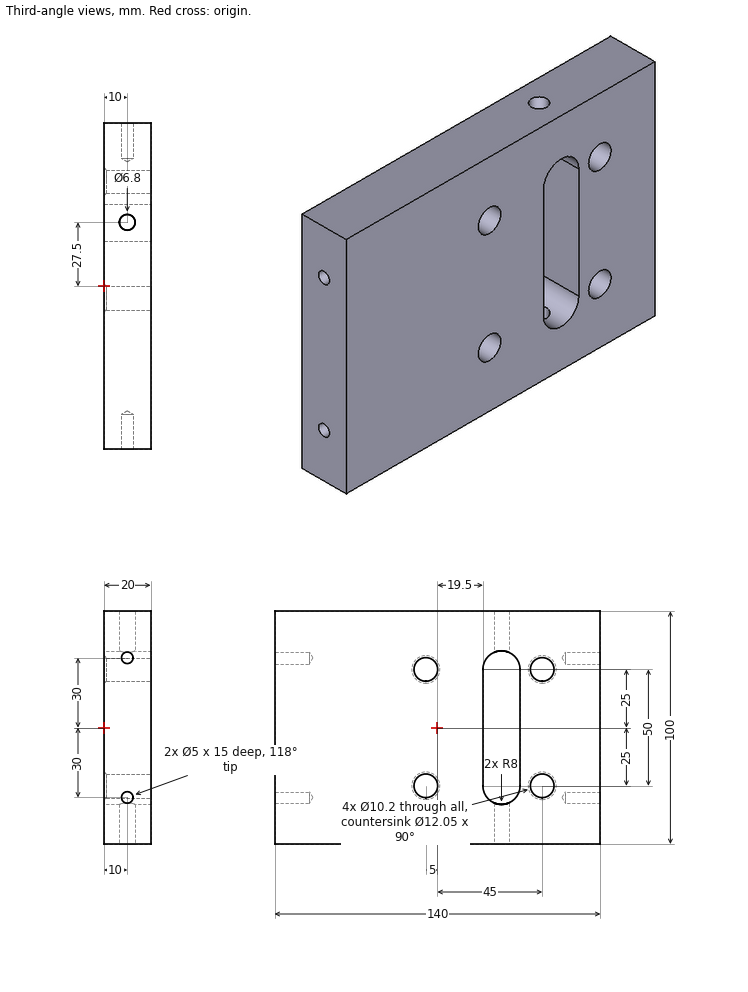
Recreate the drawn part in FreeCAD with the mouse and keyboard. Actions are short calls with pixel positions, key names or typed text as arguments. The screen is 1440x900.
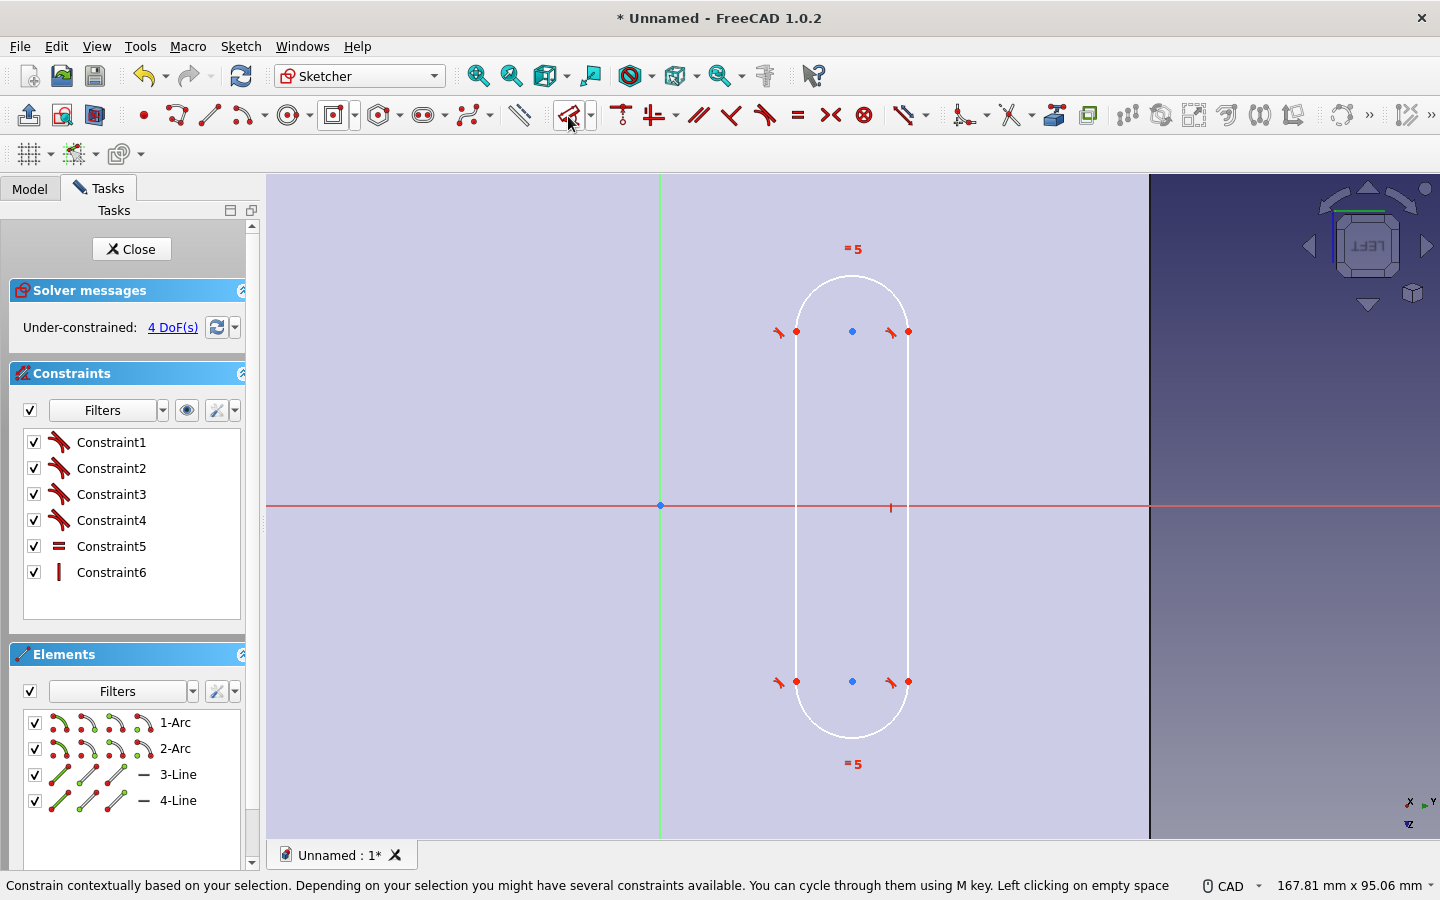
click(819, 727)
click(800, 753)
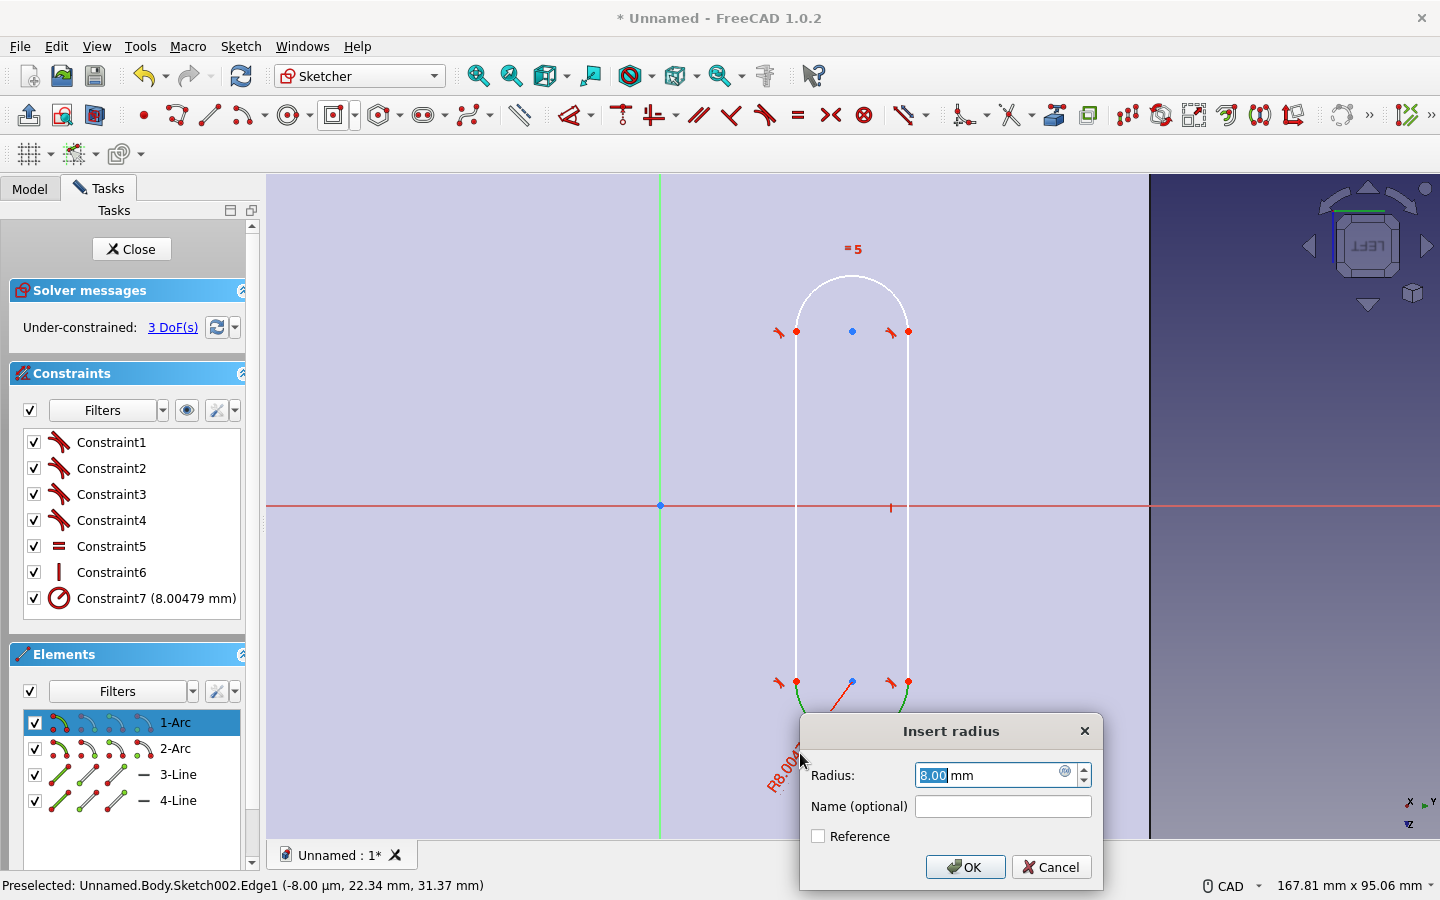
text(8)
key(Return)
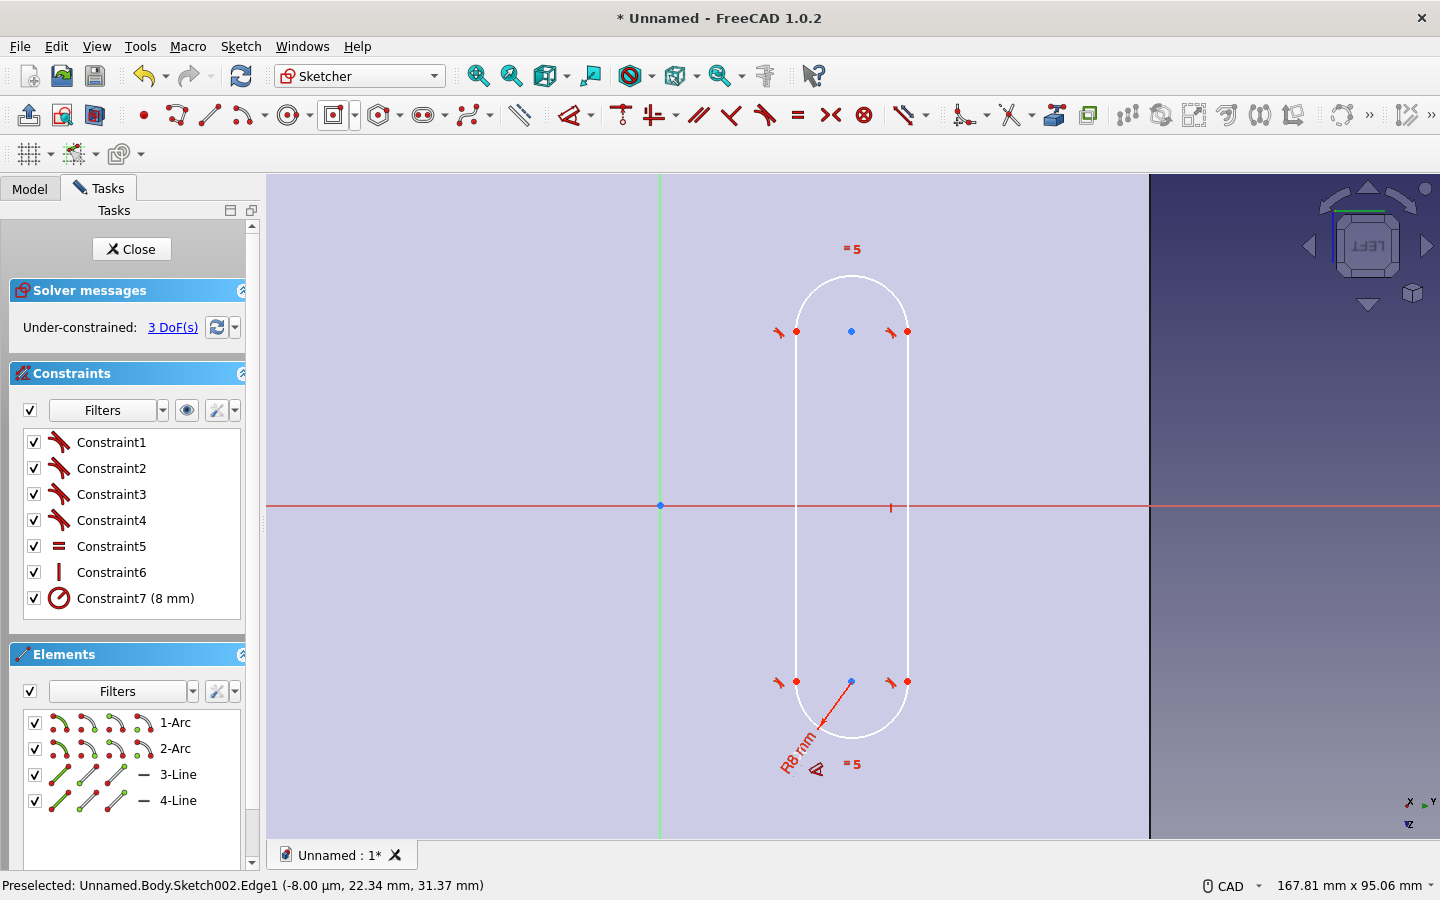
click(796, 577)
click(830, 427)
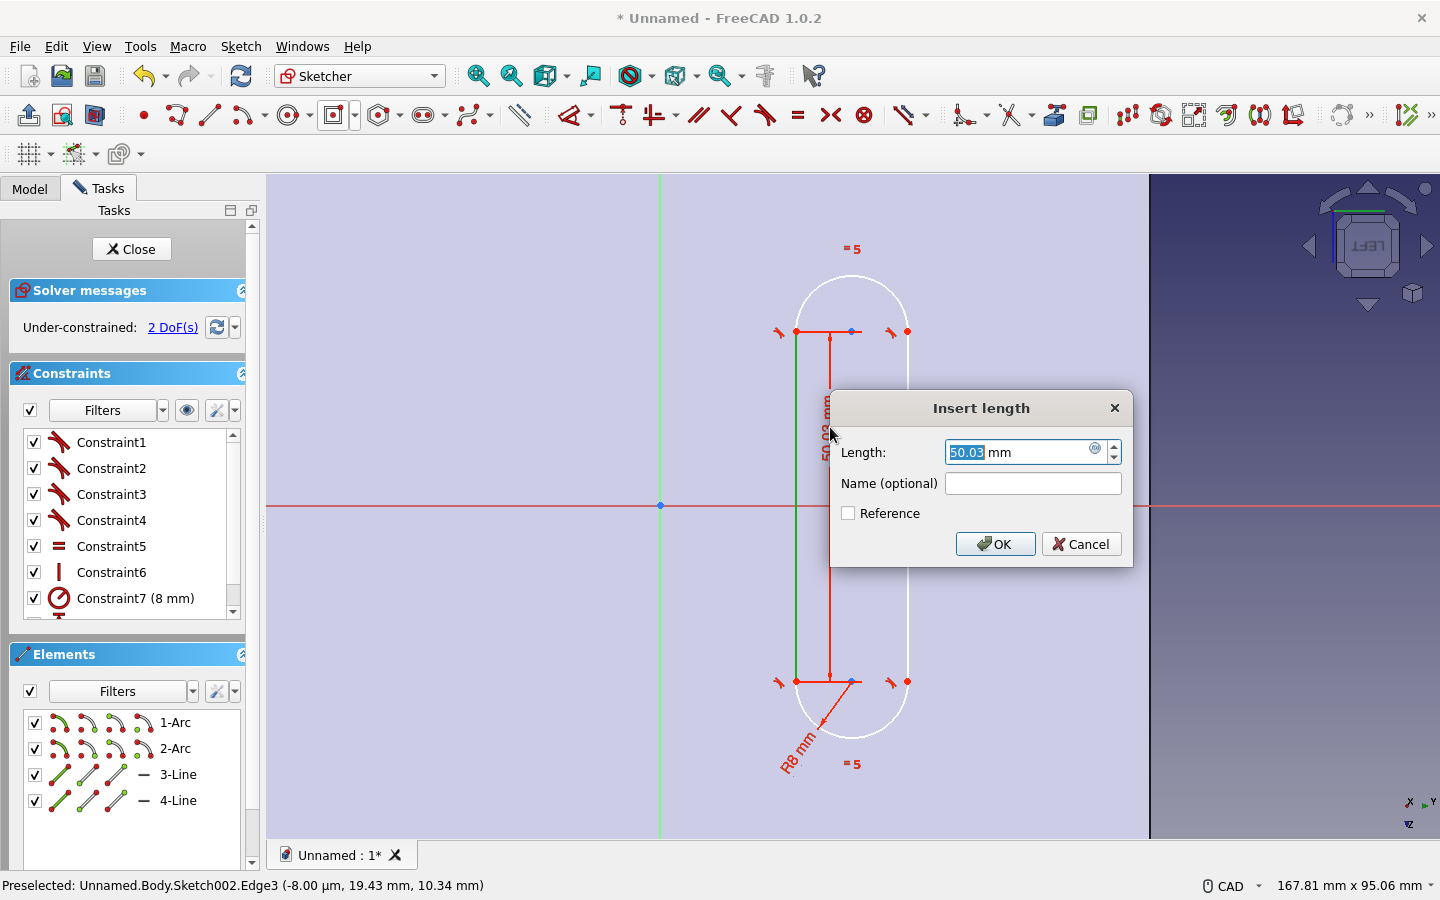
text(50)
key(Return)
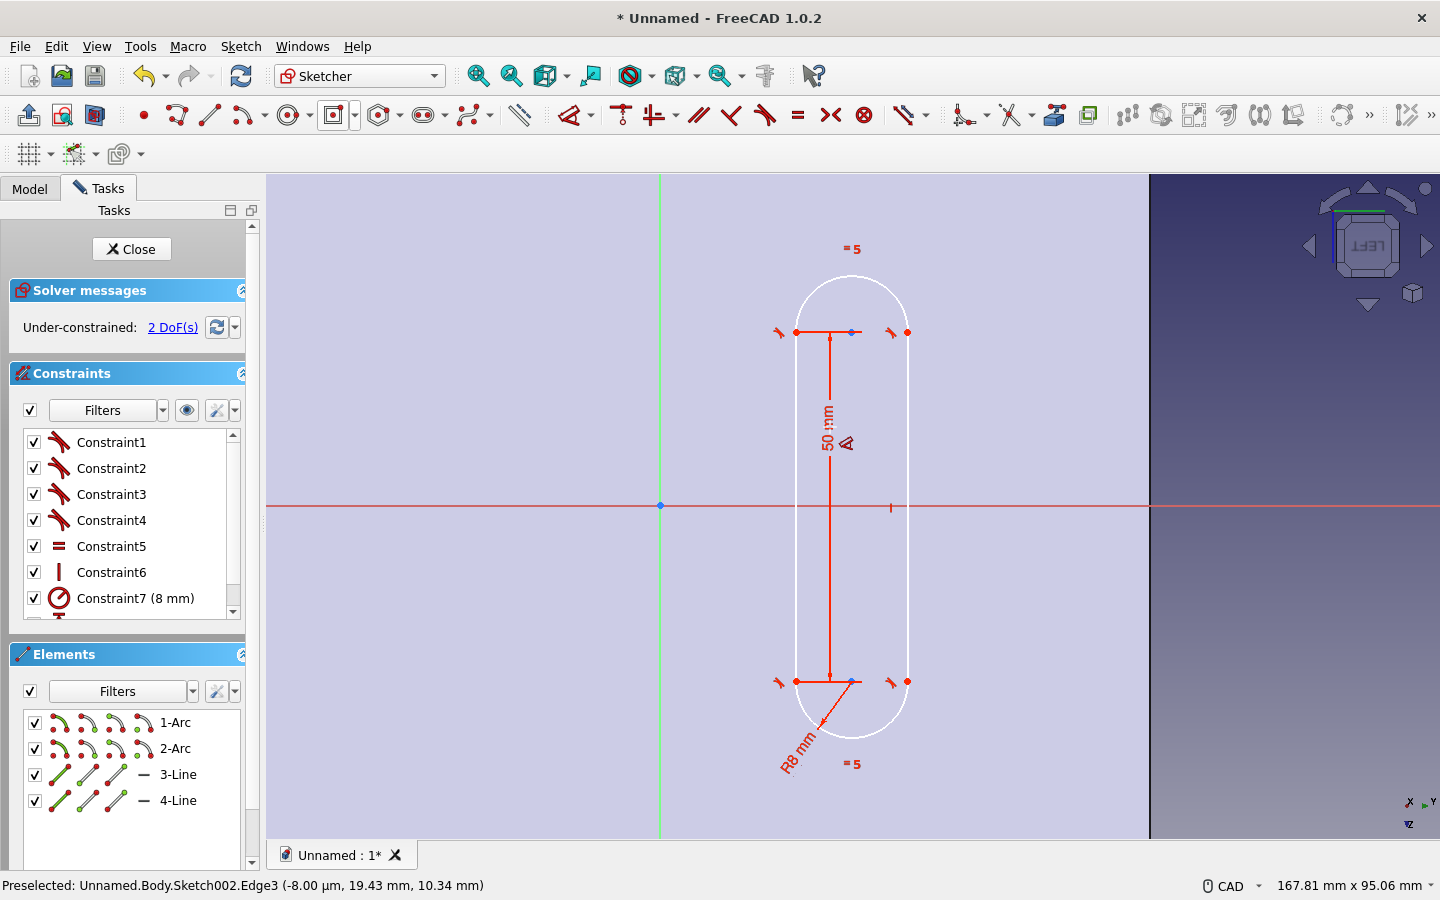
click(796, 682)
click(626, 594)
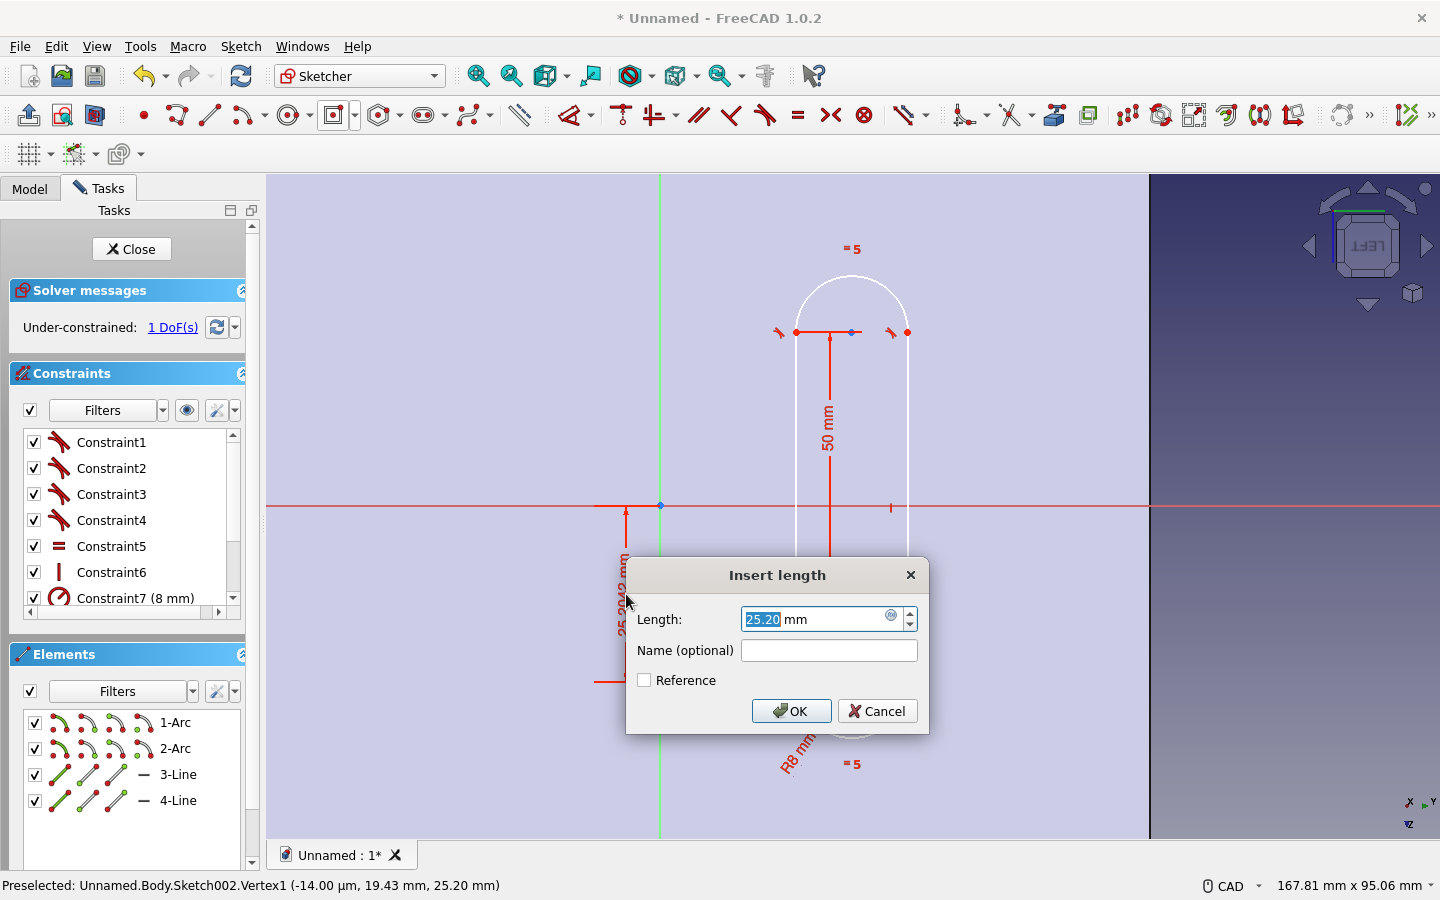
text(25)
key(Return)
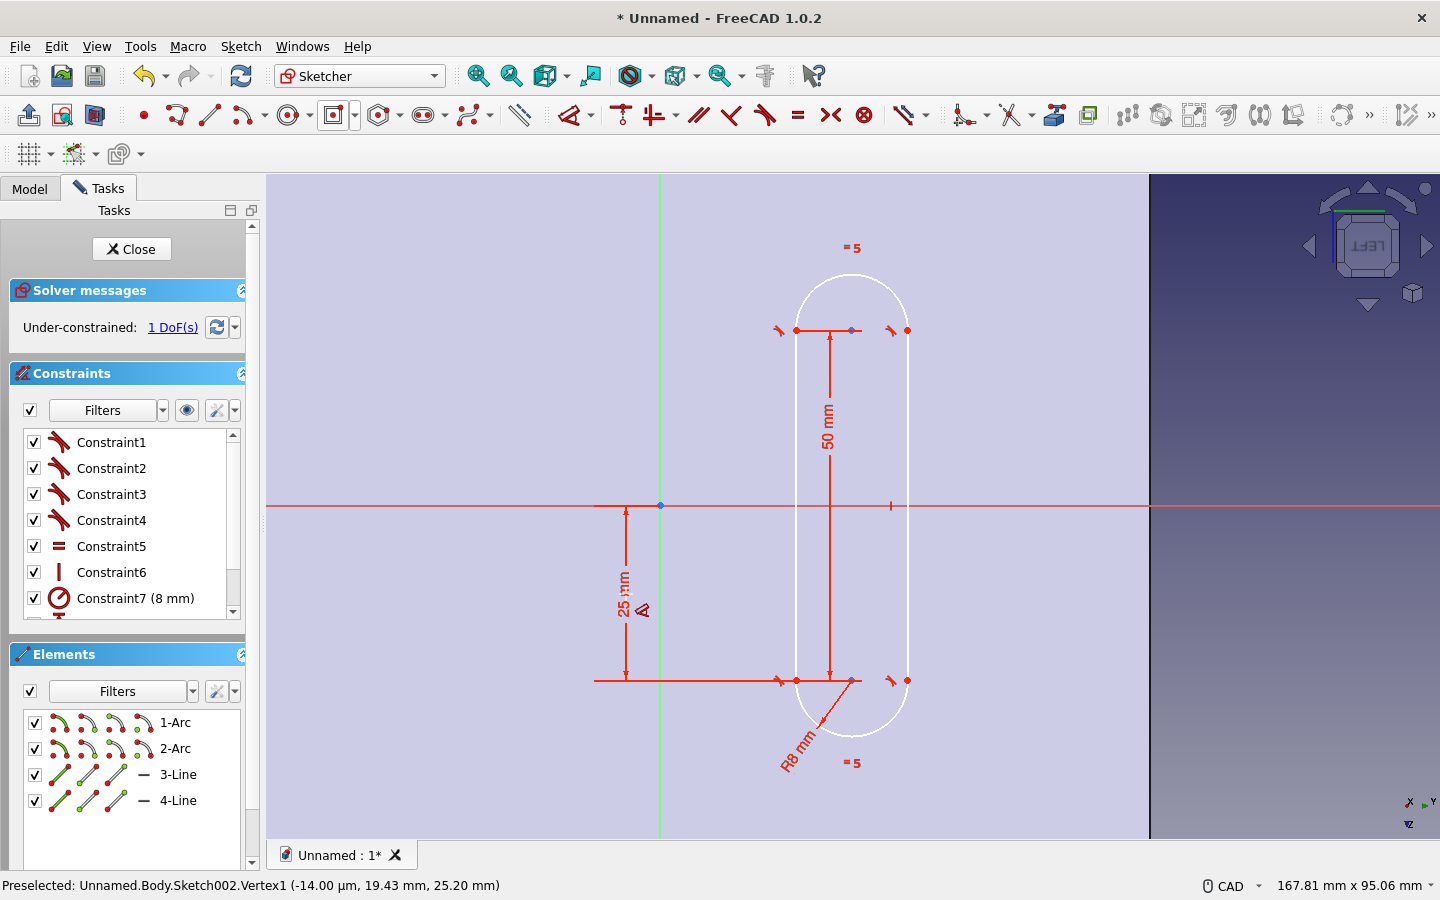
click(796, 681)
click(728, 715)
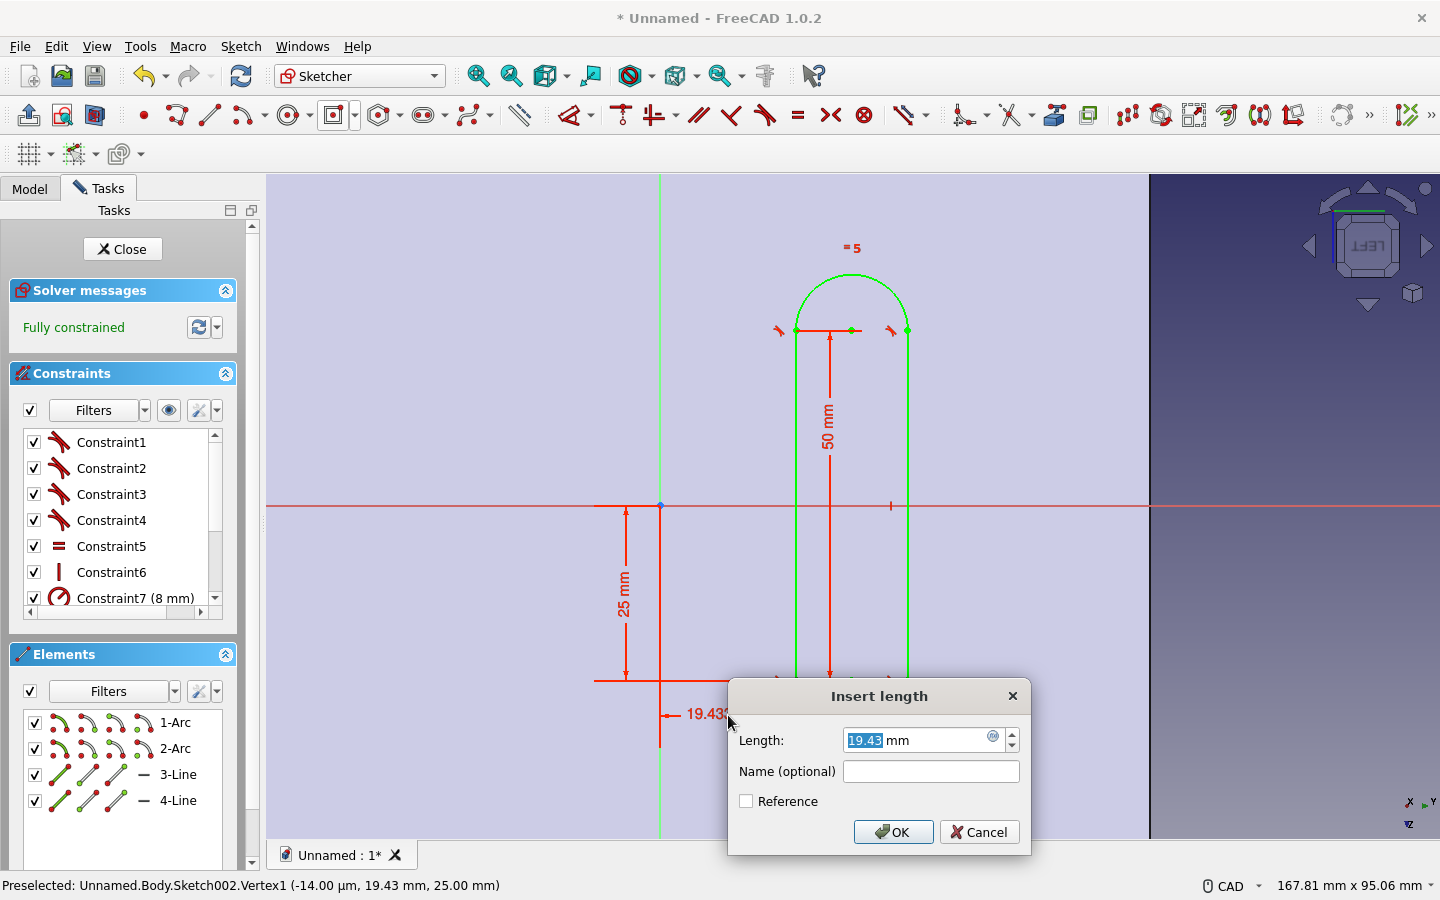
text(19.5)
key(Return)
key(Escape)